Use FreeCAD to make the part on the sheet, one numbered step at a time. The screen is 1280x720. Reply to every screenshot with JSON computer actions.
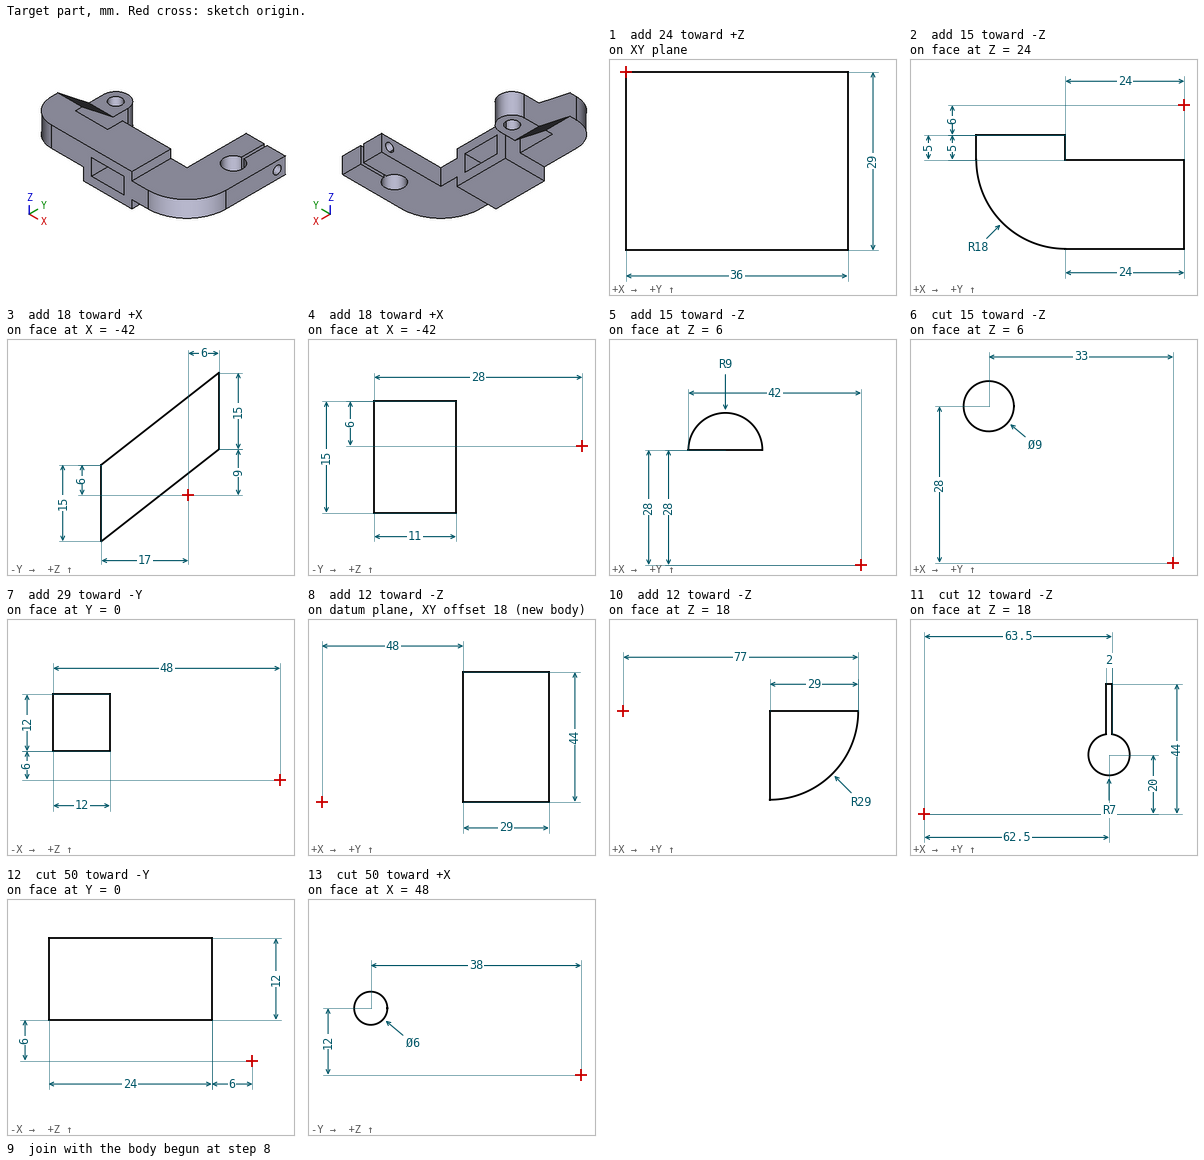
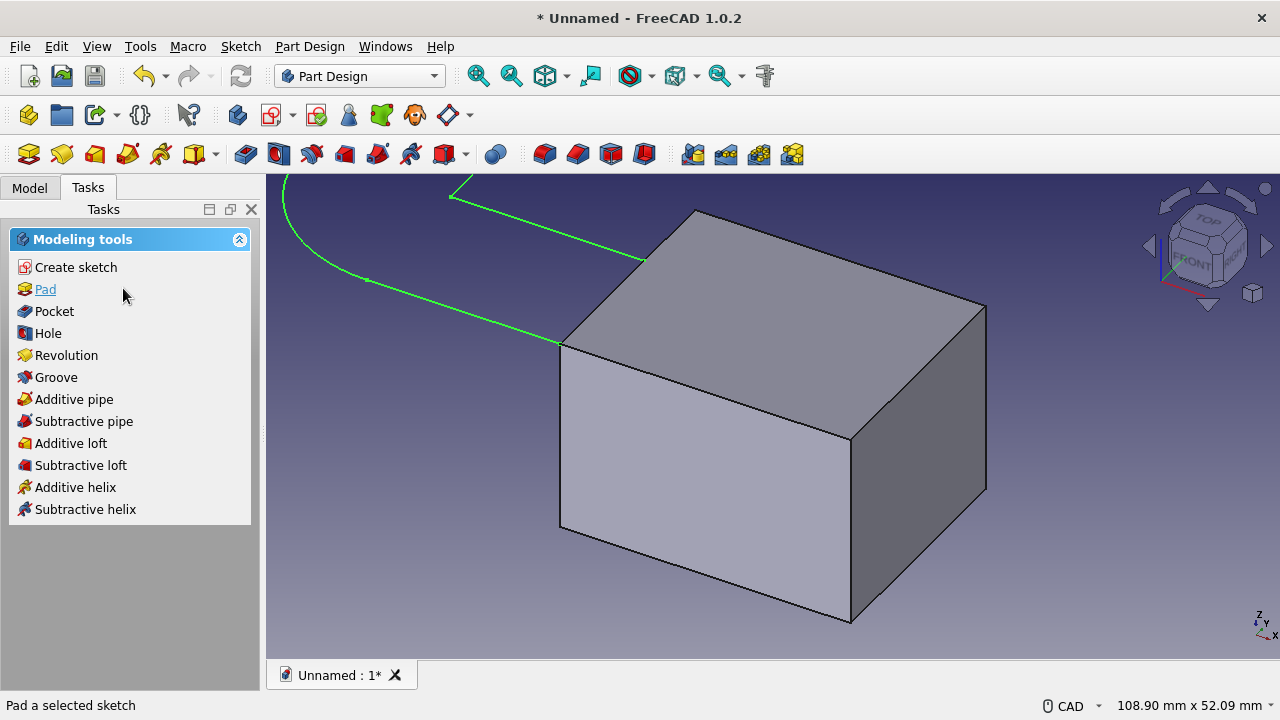
{"action": "left_click", "coordinate": [29, 154]}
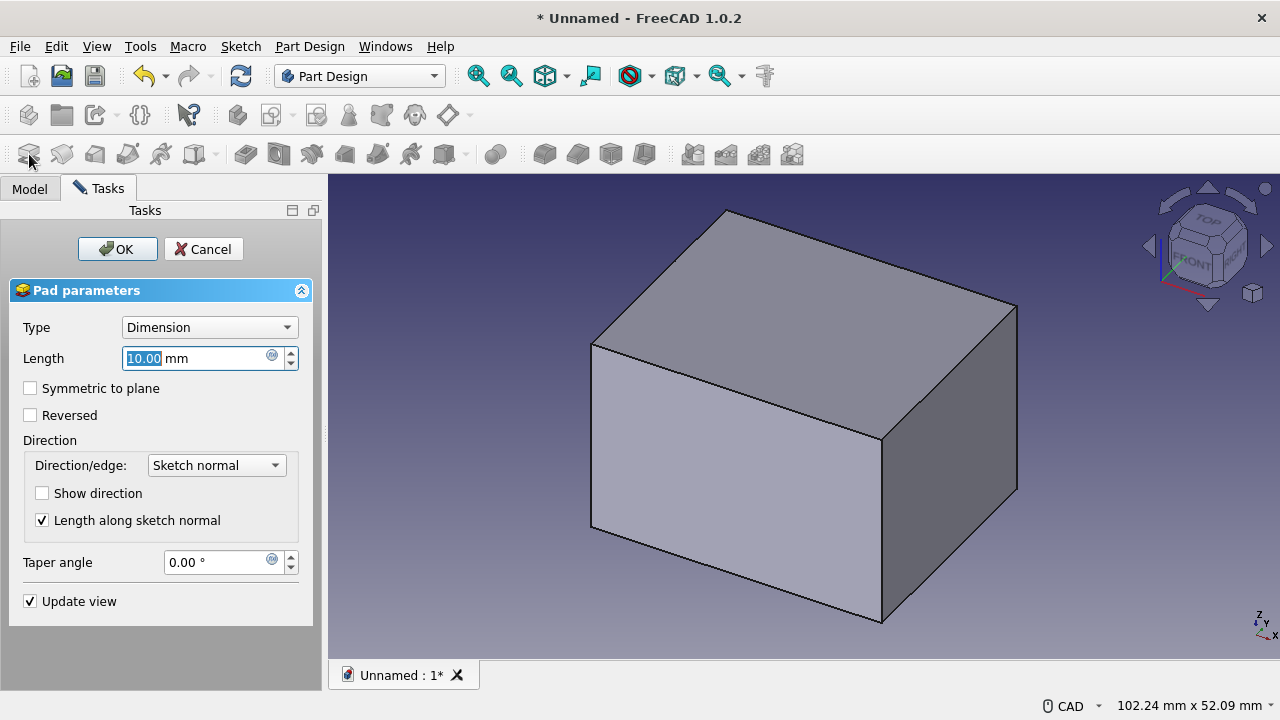
{"action": "type", "text": "15"}
{"action": "key", "text": "Tab"}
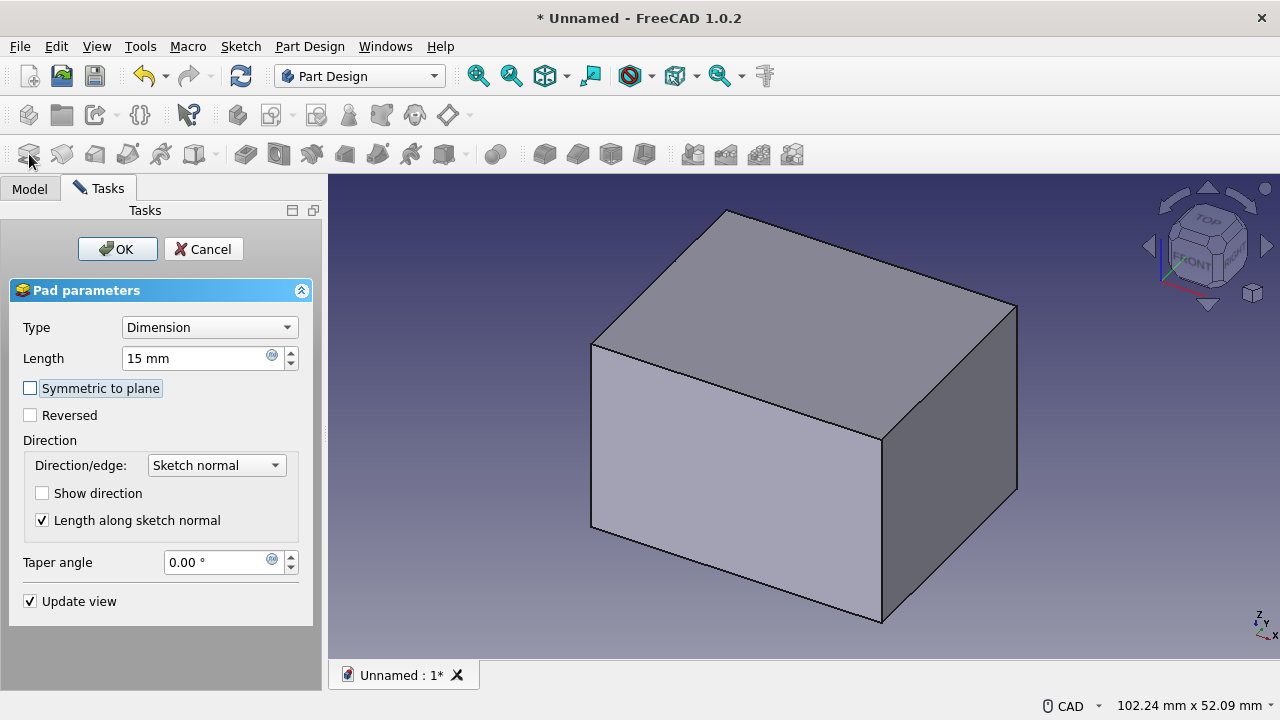
{"action": "left_click", "coordinate": [31, 415]}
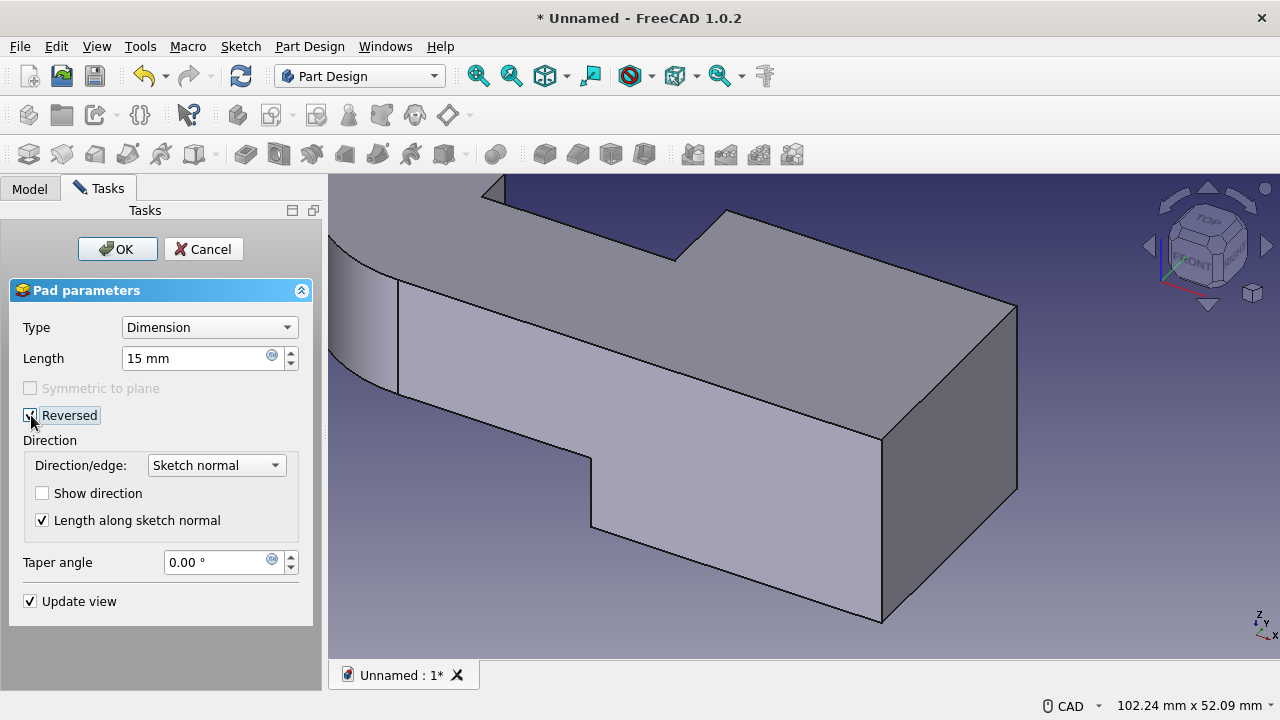
{"action": "left_click", "coordinate": [118, 249]}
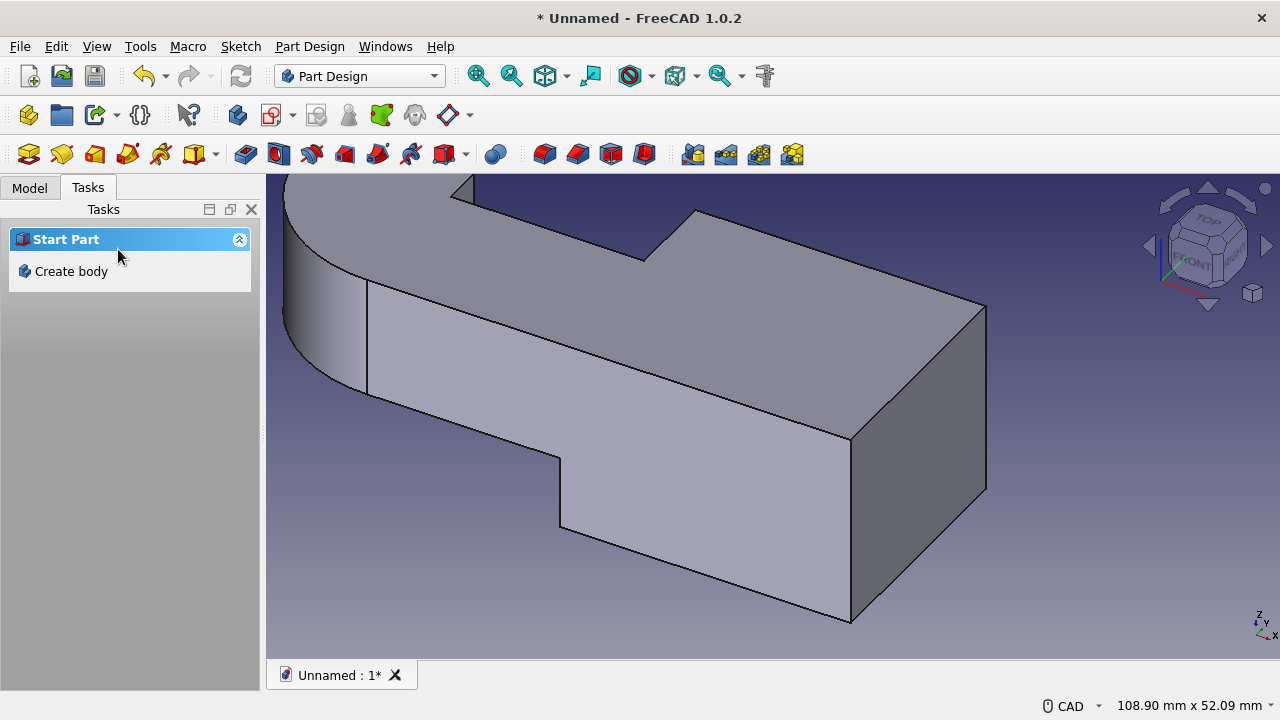
{"action": "left_click", "coordinate": [479, 76]}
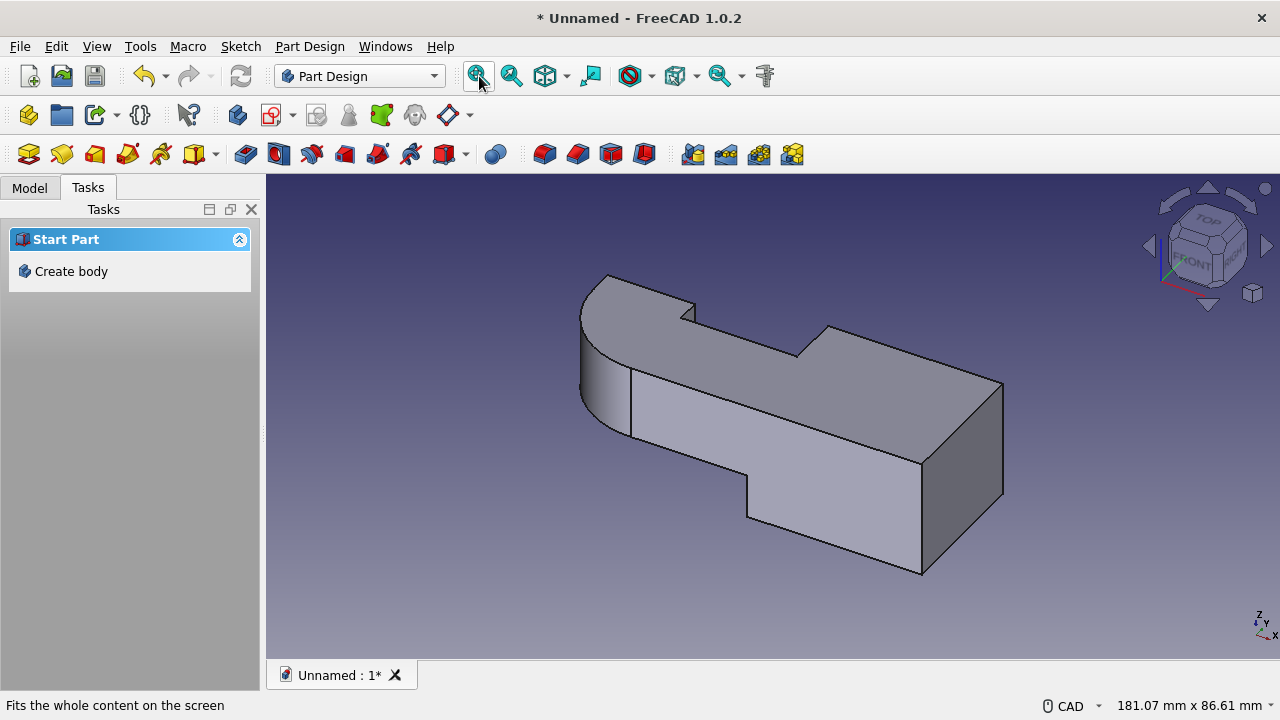
{"action": "key", "text": "6"}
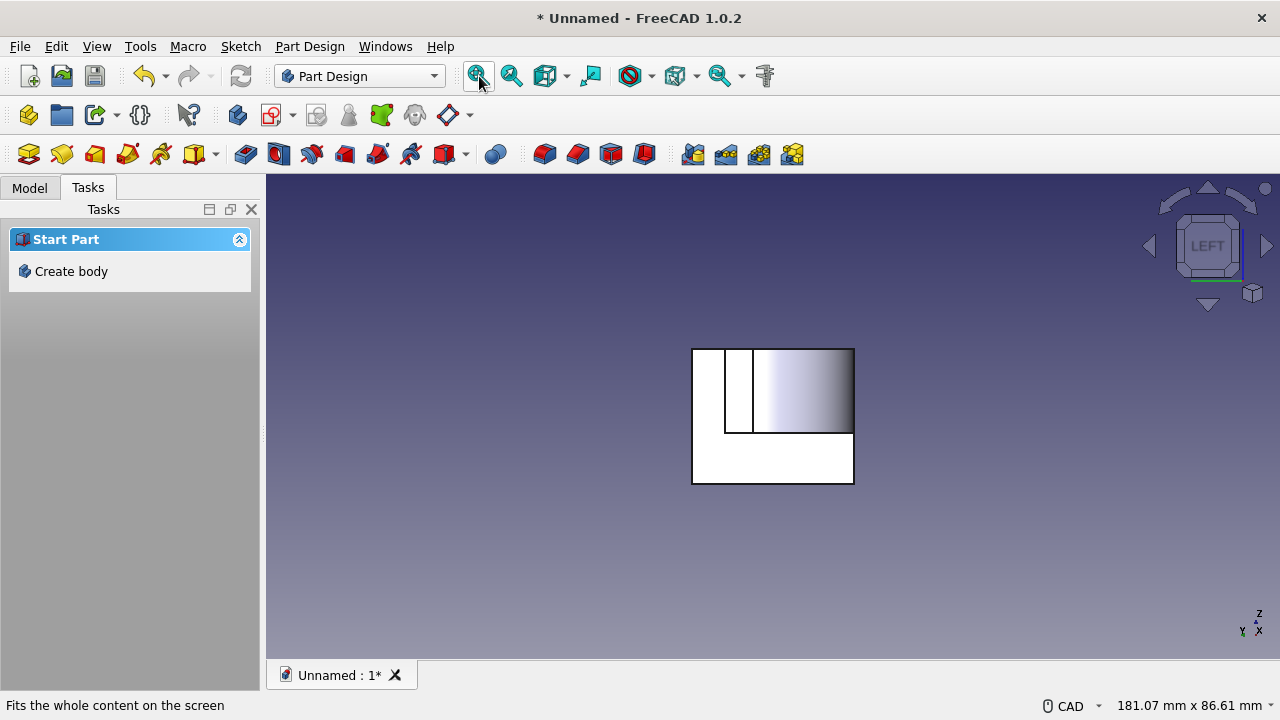
{"action": "key", "text": "v f"}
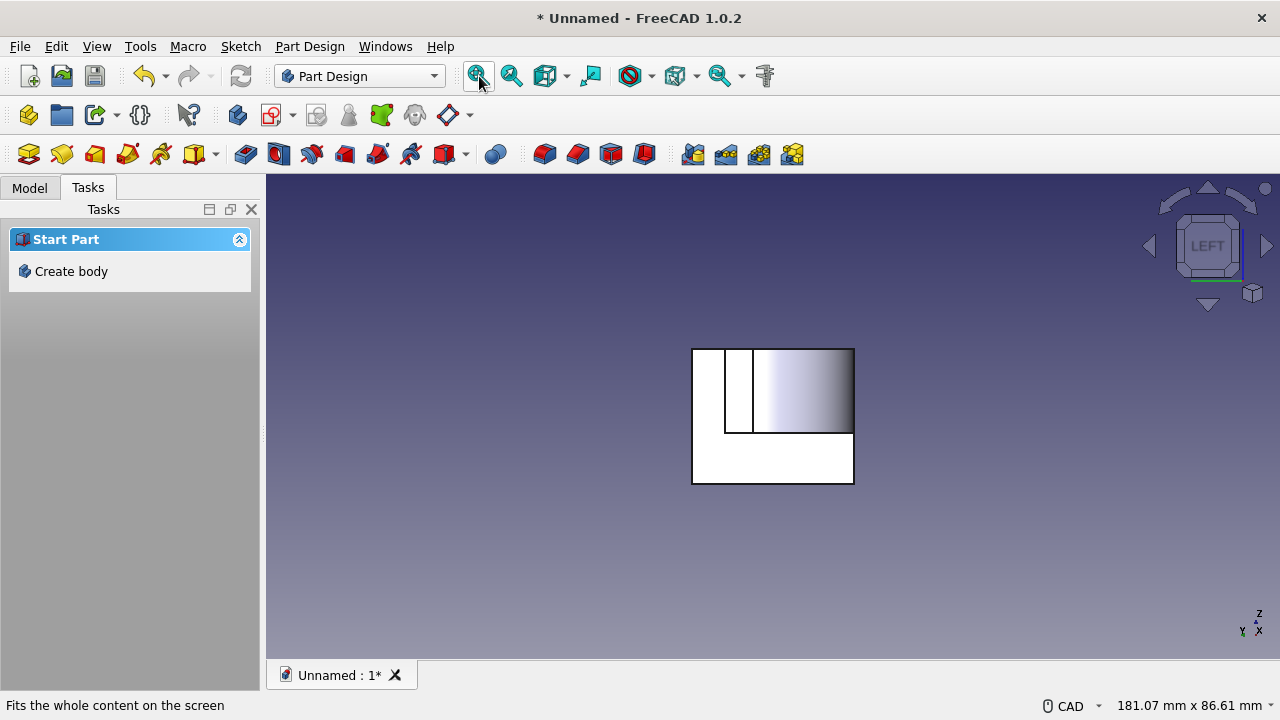
{"action": "left_click", "coordinate": [739, 366]}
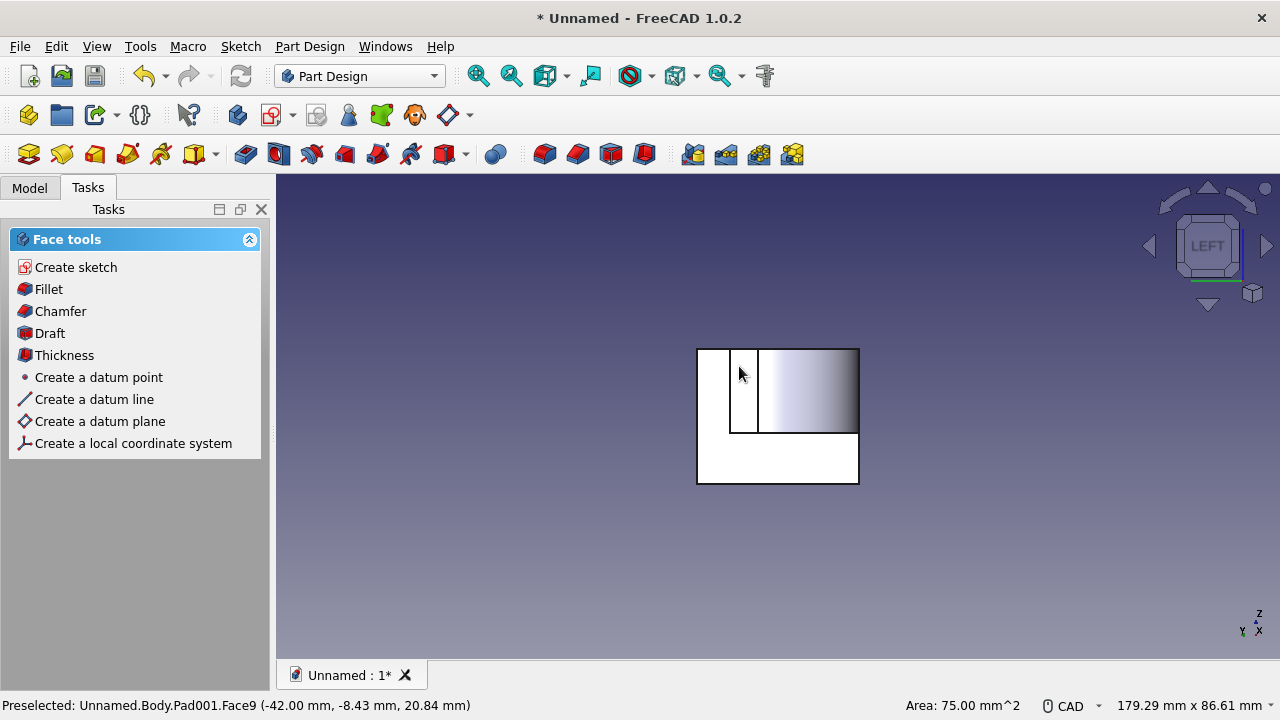
{"action": "left_click", "coordinate": [270, 116]}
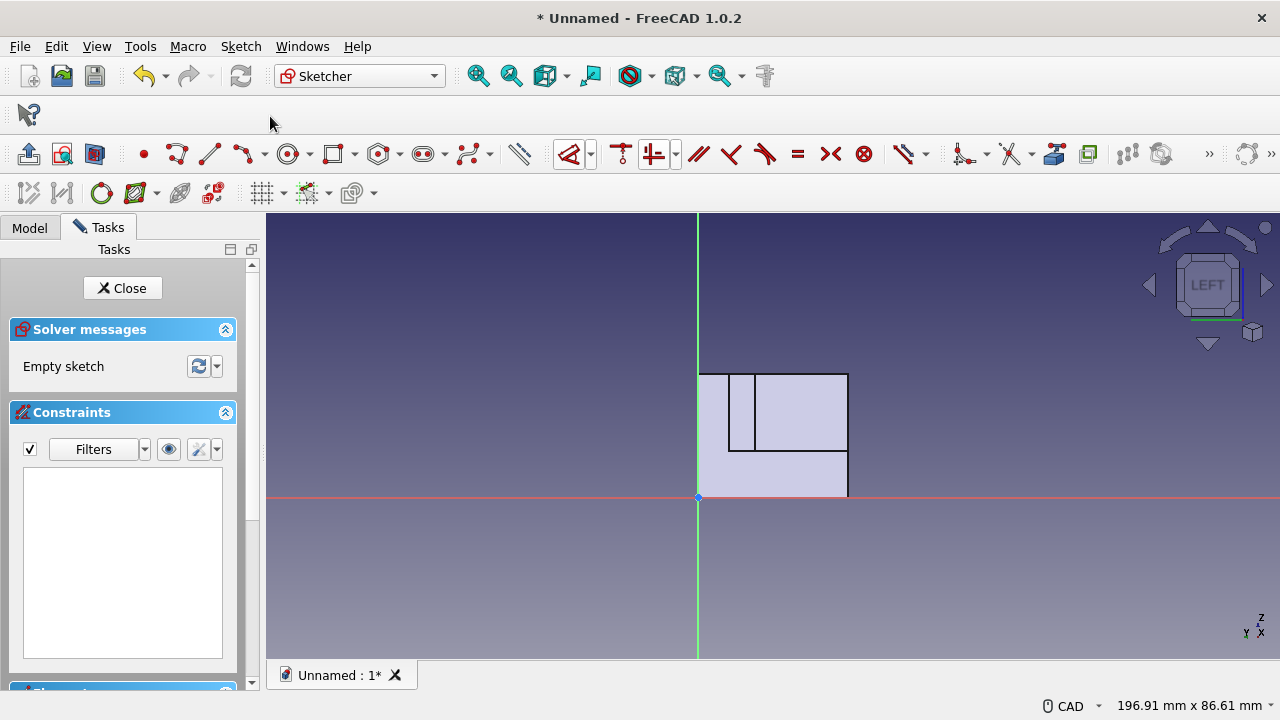
{"action": "scroll", "coordinate": [600, 506], "scroll_direction": "up", "scroll_amount": 2}